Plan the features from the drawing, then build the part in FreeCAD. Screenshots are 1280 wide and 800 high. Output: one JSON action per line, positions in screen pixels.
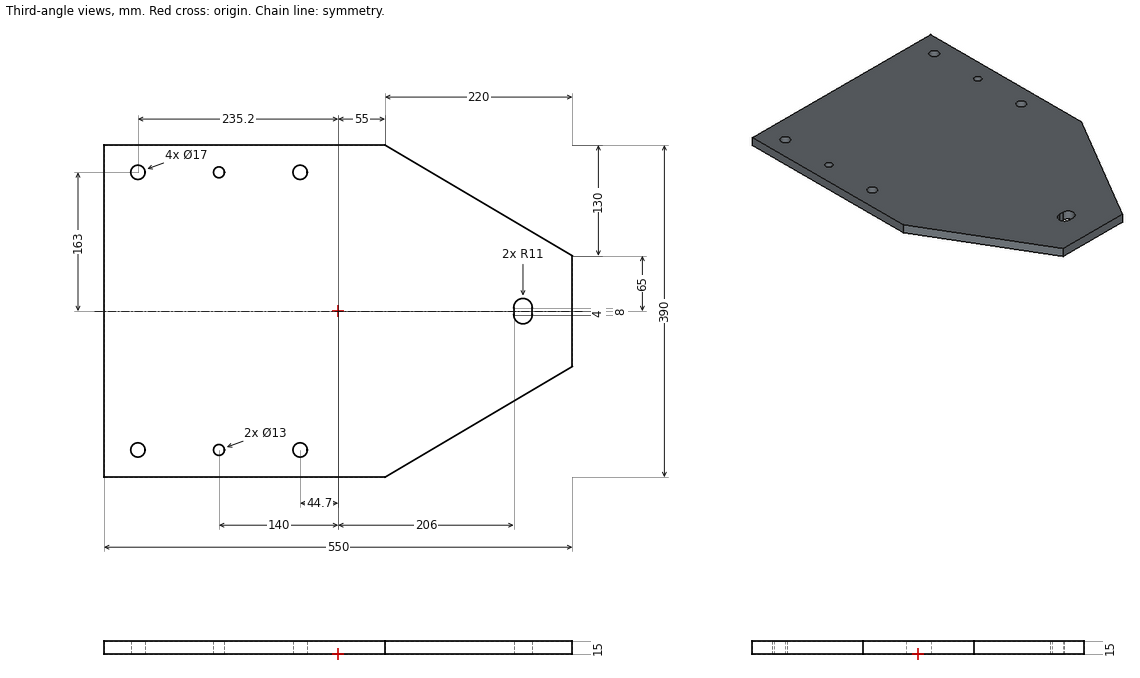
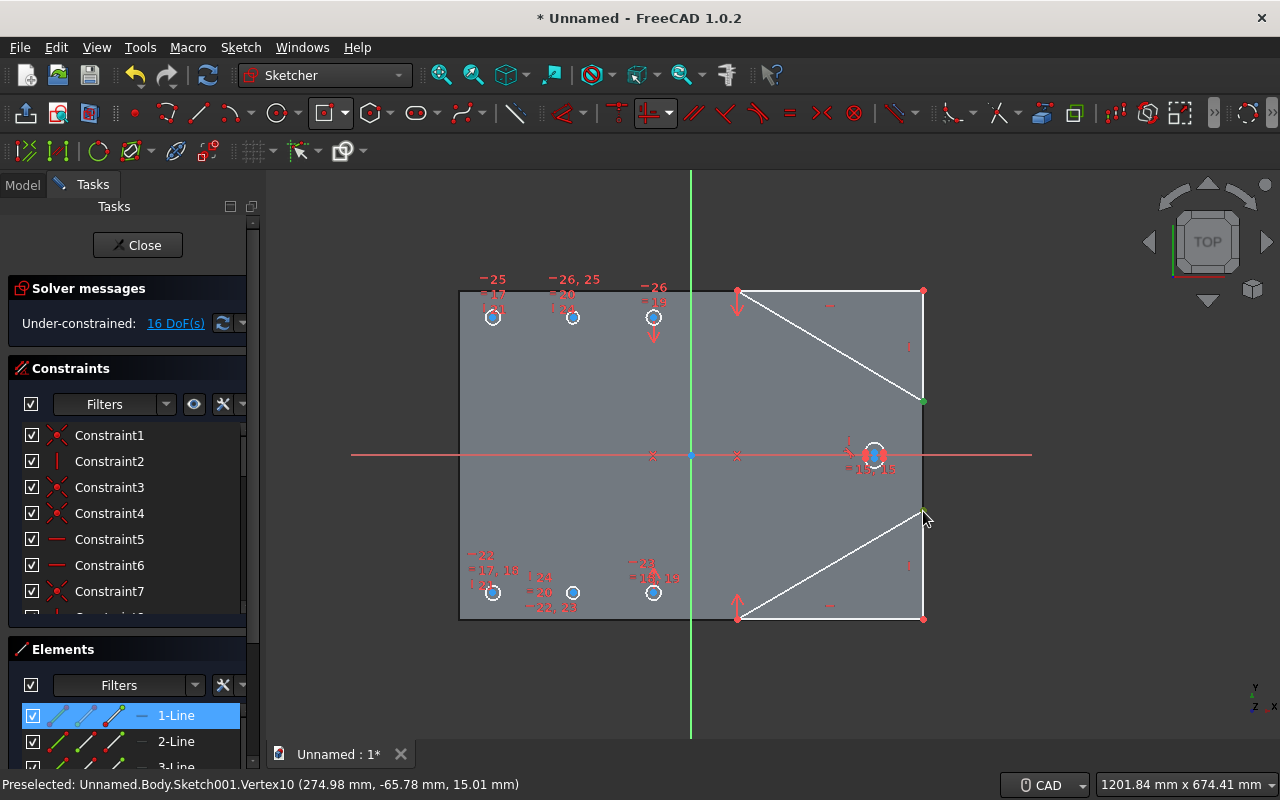
{"action": "left_click", "coordinate": [353, 455]}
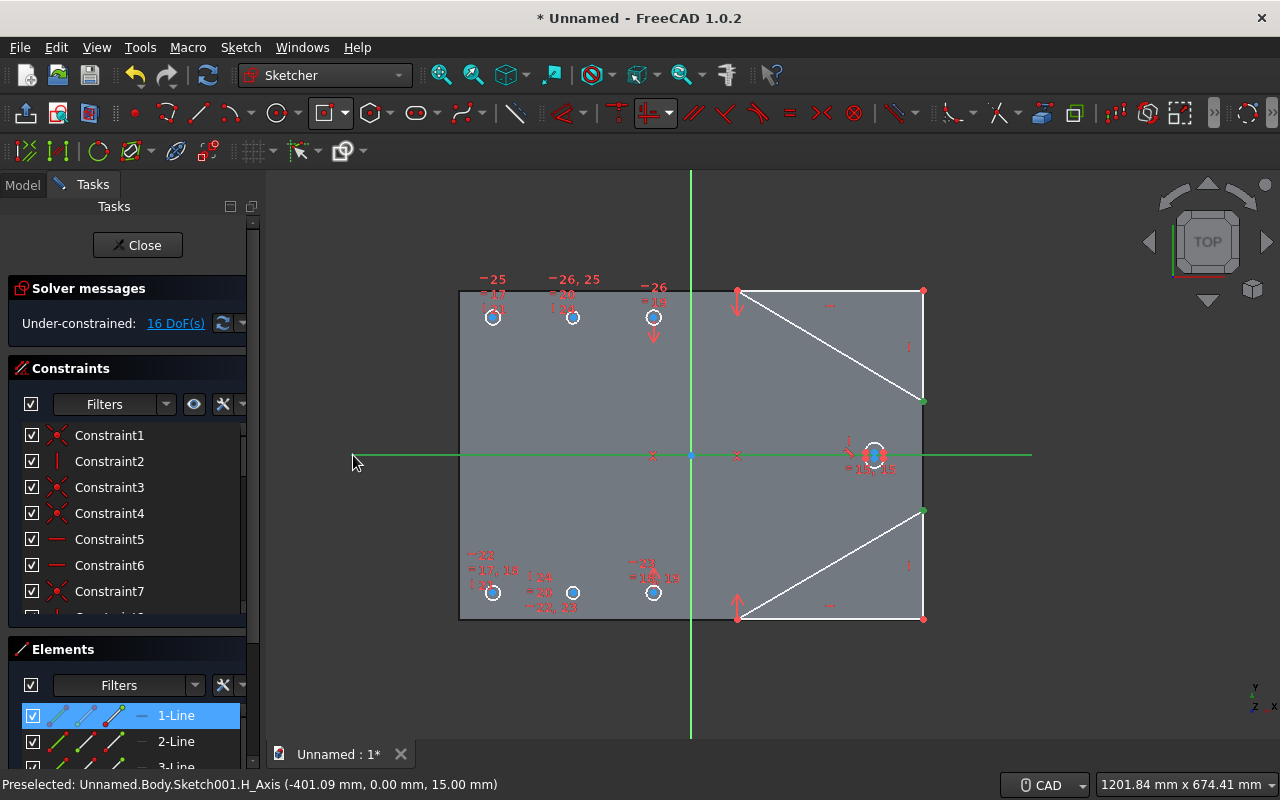
{"action": "left_click", "coordinate": [822, 114]}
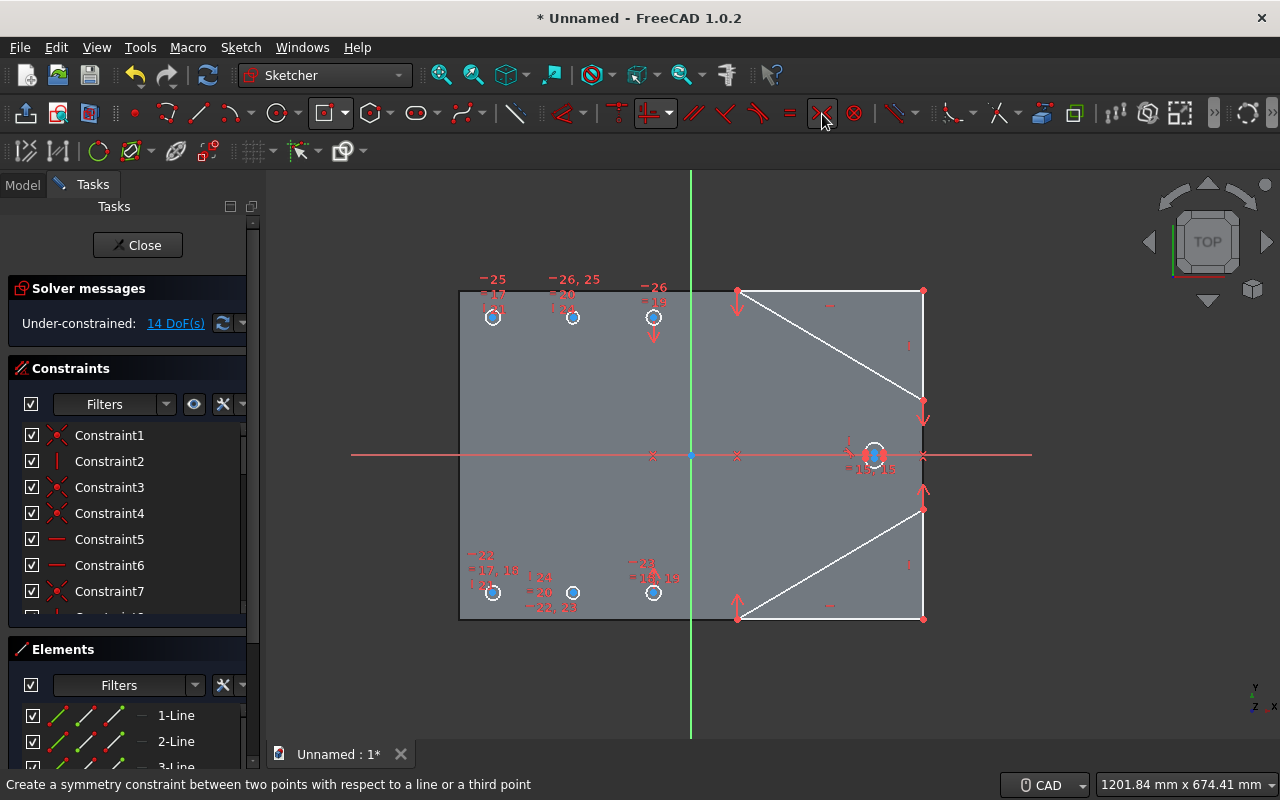
{"action": "left_click", "coordinate": [562, 114]}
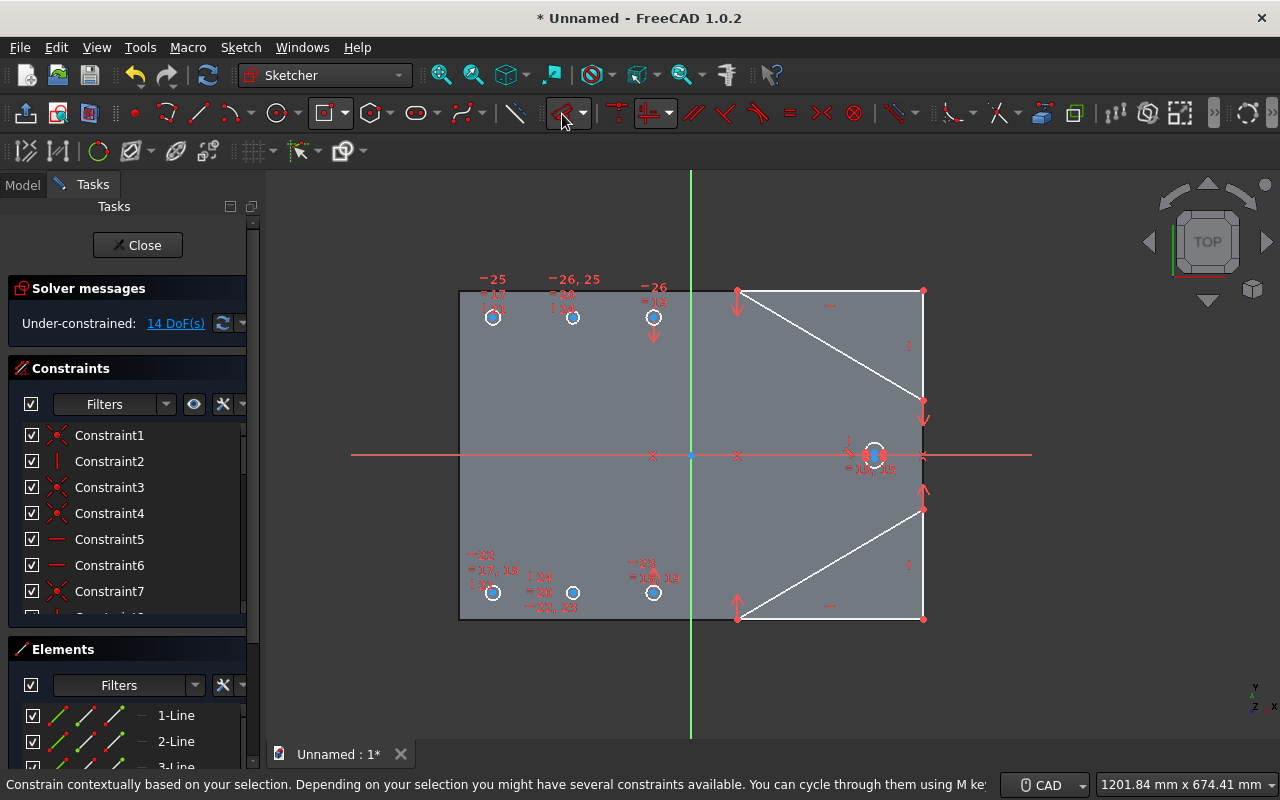
{"action": "scroll", "coordinate": [875, 468], "scroll_direction": "up", "scroll_amount": 8}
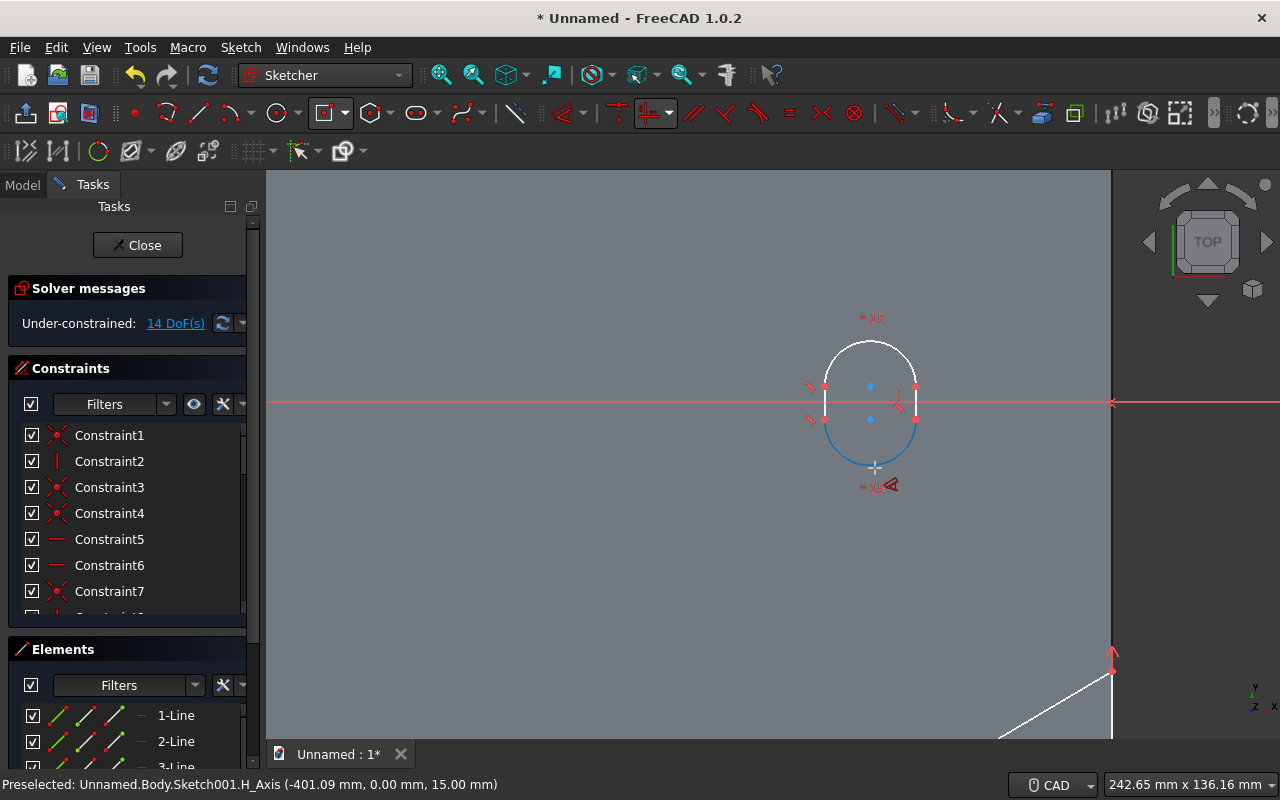
{"action": "left_click", "coordinate": [870, 465]}
{"action": "left_click", "coordinate": [870, 497]}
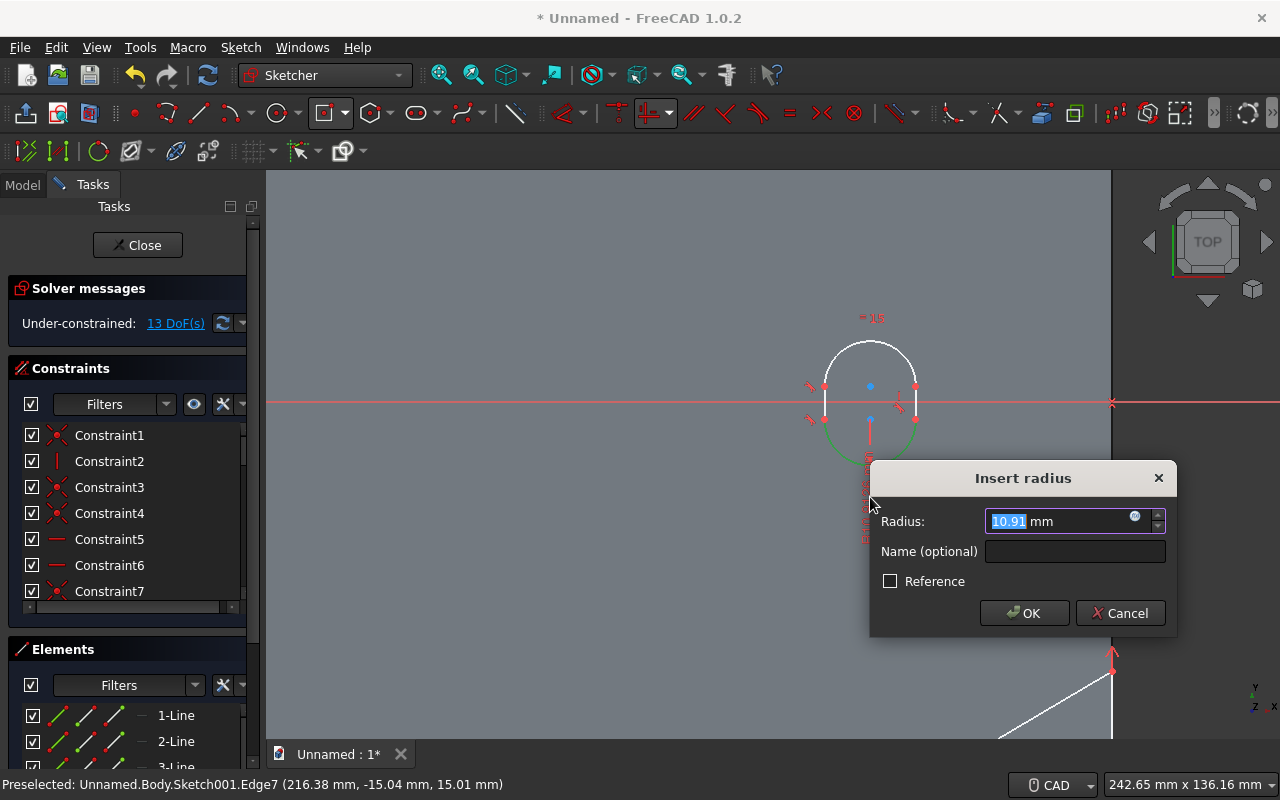
{"action": "type", "text": "11"}
{"action": "key", "text": "Return"}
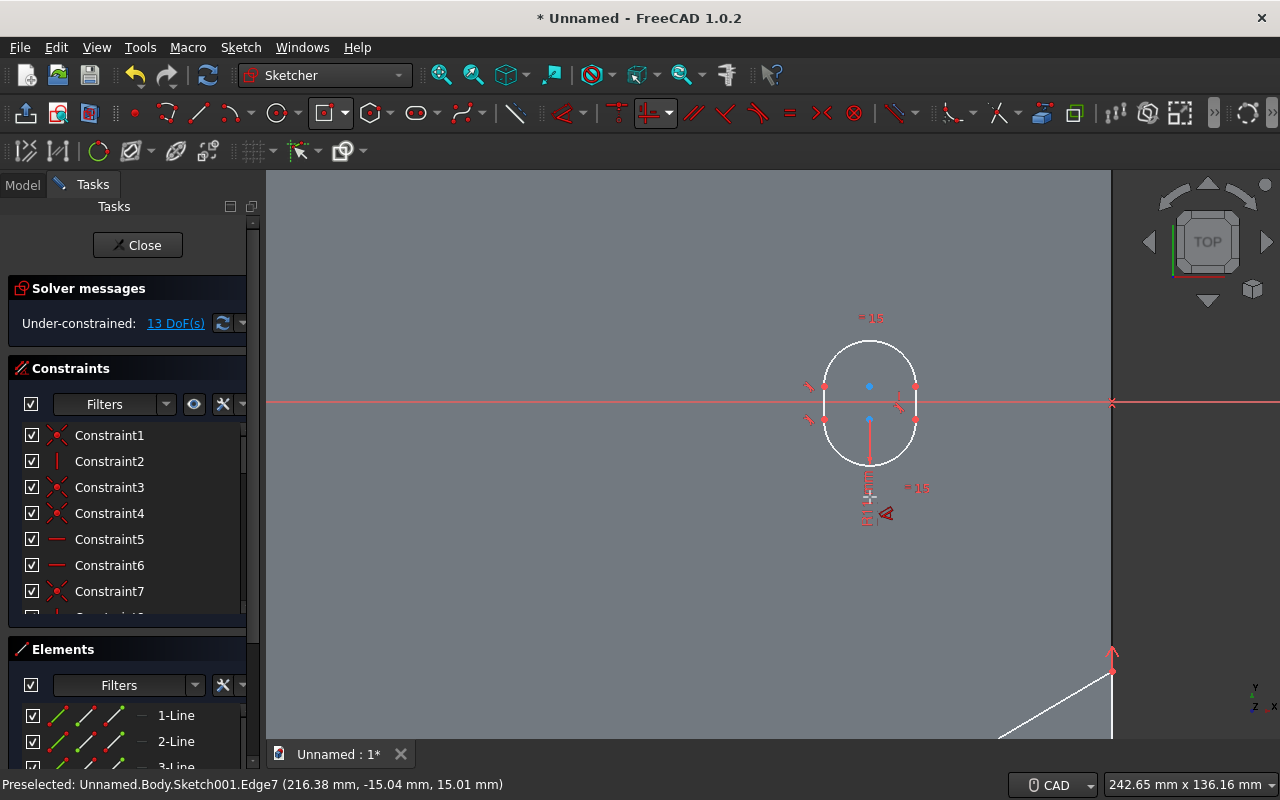
{"action": "scroll", "coordinate": [875, 468], "scroll_direction": "down", "scroll_amount": 8}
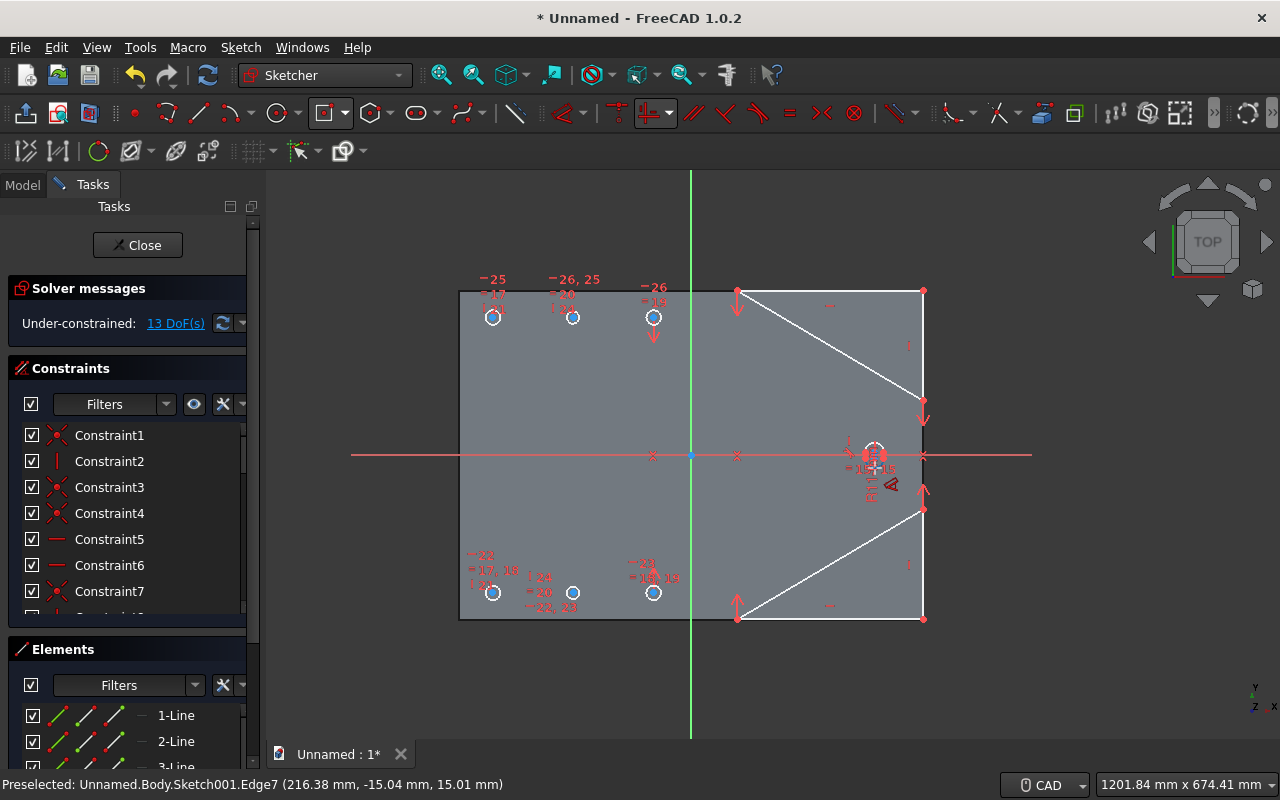
{"action": "scroll", "coordinate": [498, 312], "scroll_direction": "up", "scroll_amount": 6}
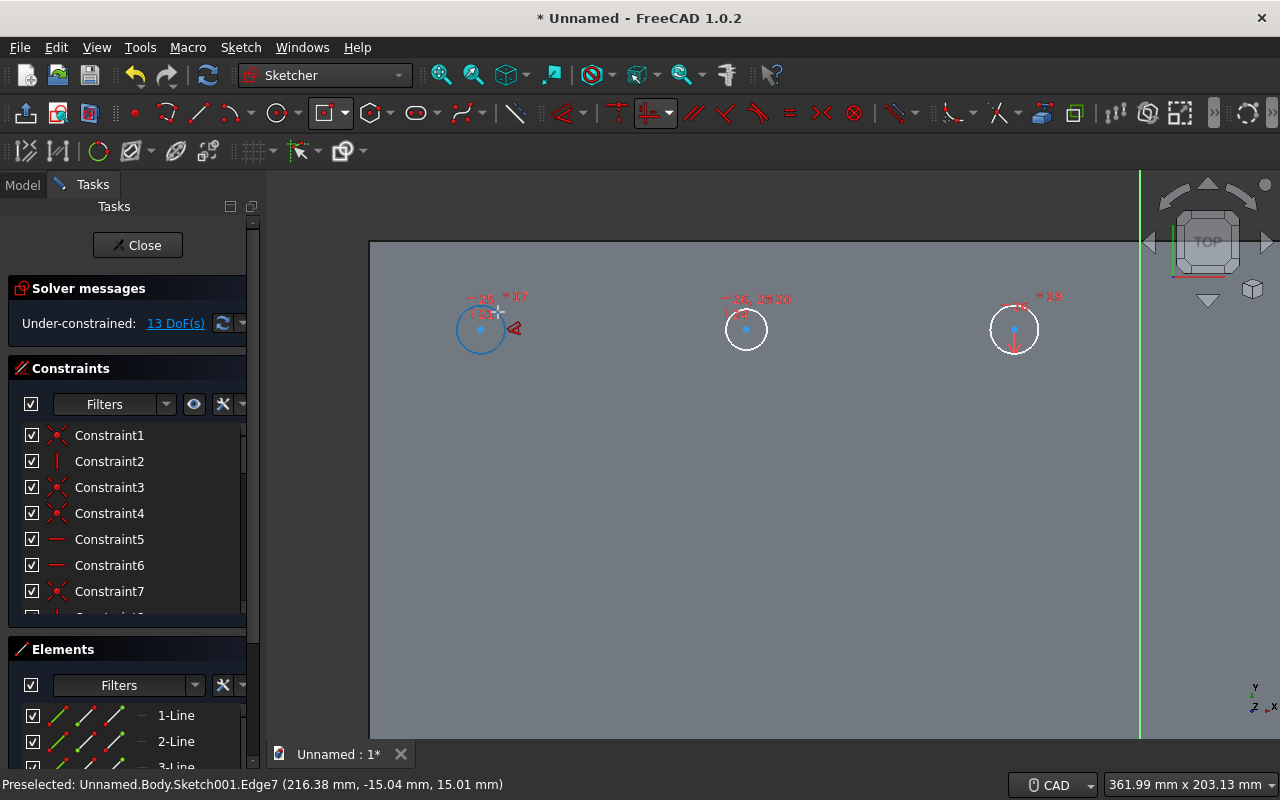
{"action": "left_click", "coordinate": [498, 313]}
{"action": "left_click", "coordinate": [521, 291]}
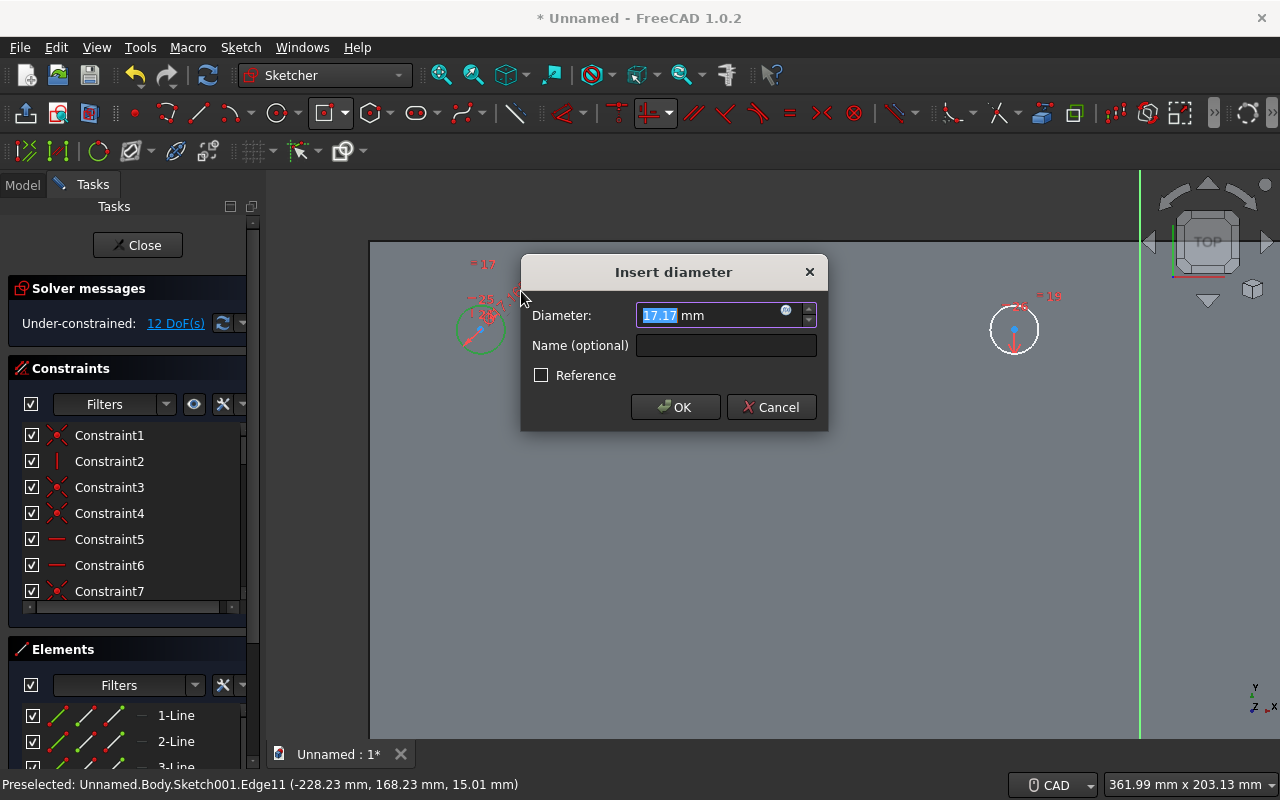
{"action": "type", "text": "17"}
{"action": "key", "text": "Return"}